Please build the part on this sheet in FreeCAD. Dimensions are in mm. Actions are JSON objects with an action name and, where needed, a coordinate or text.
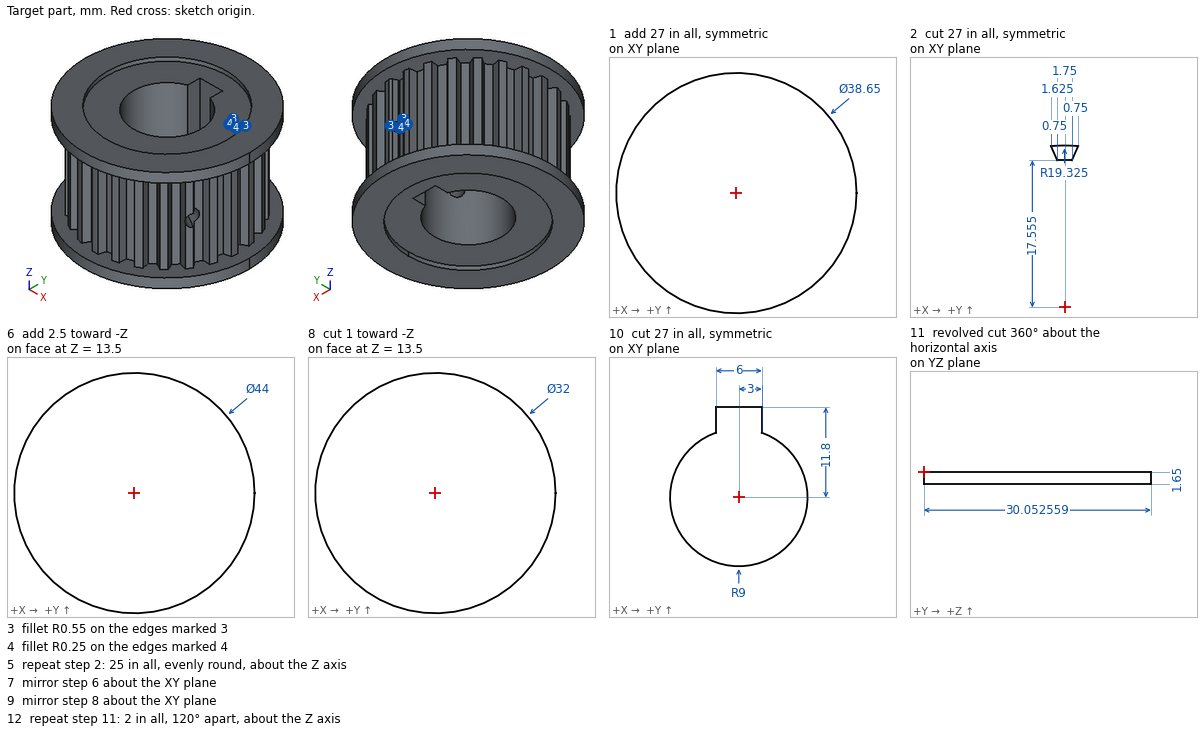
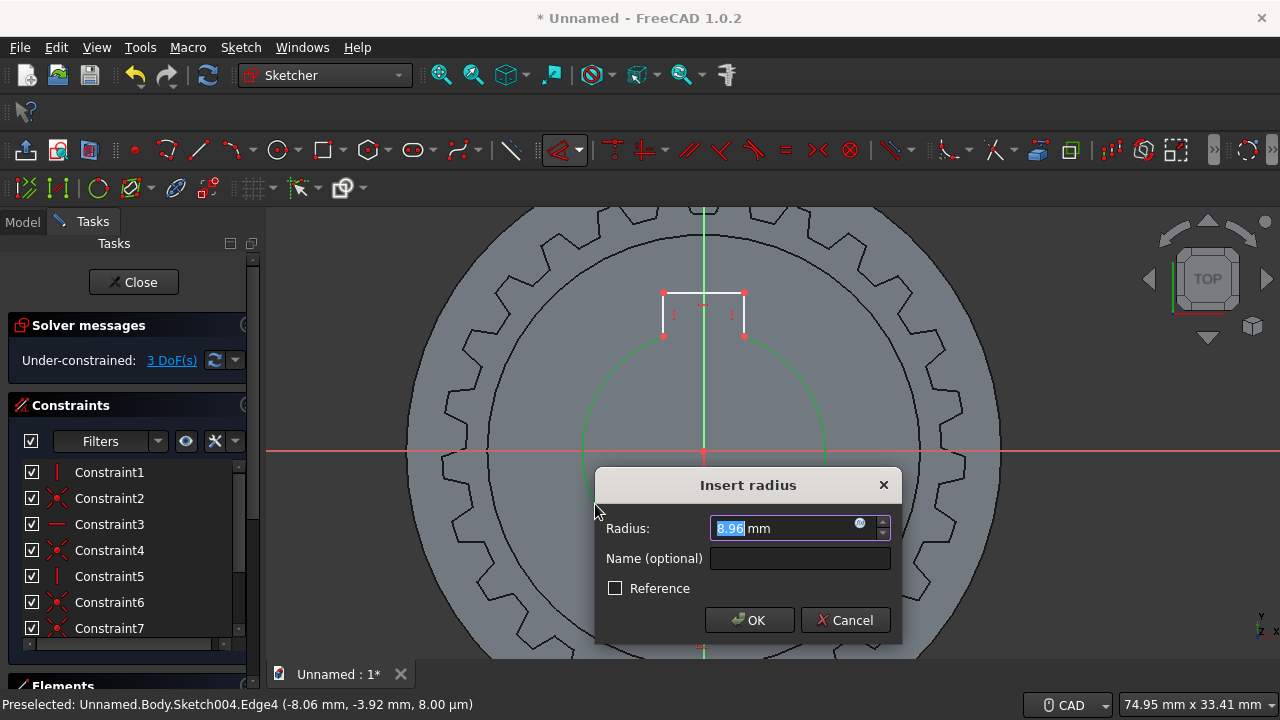
{"action": "type", "text": "9"}
{"action": "key", "text": "Return"}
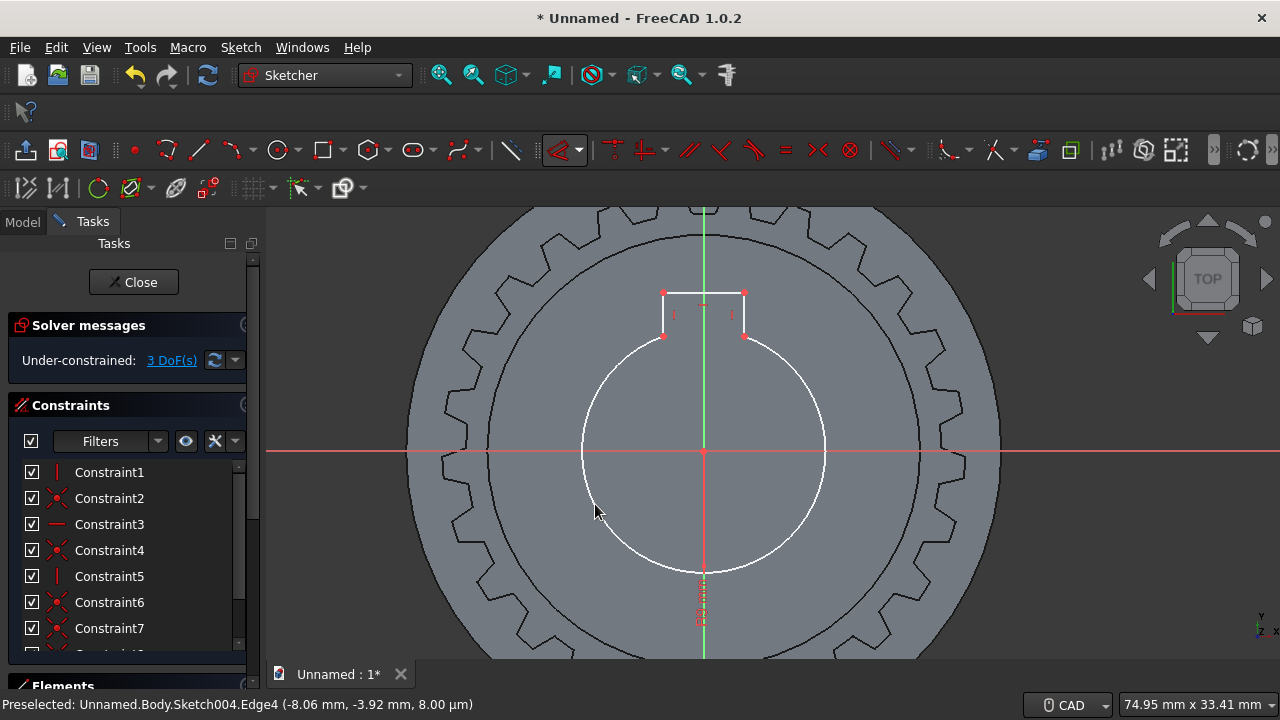
{"action": "left_click", "coordinate": [720, 293]}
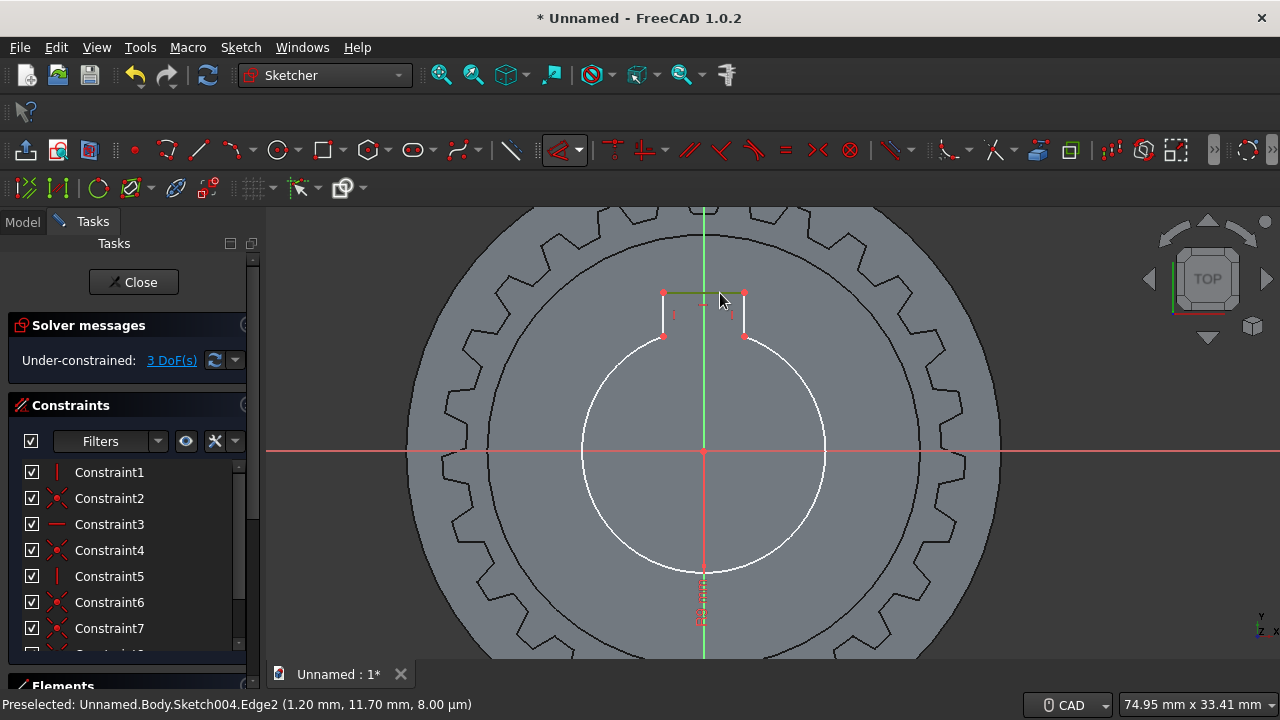
{"action": "left_click", "coordinate": [582, 150]}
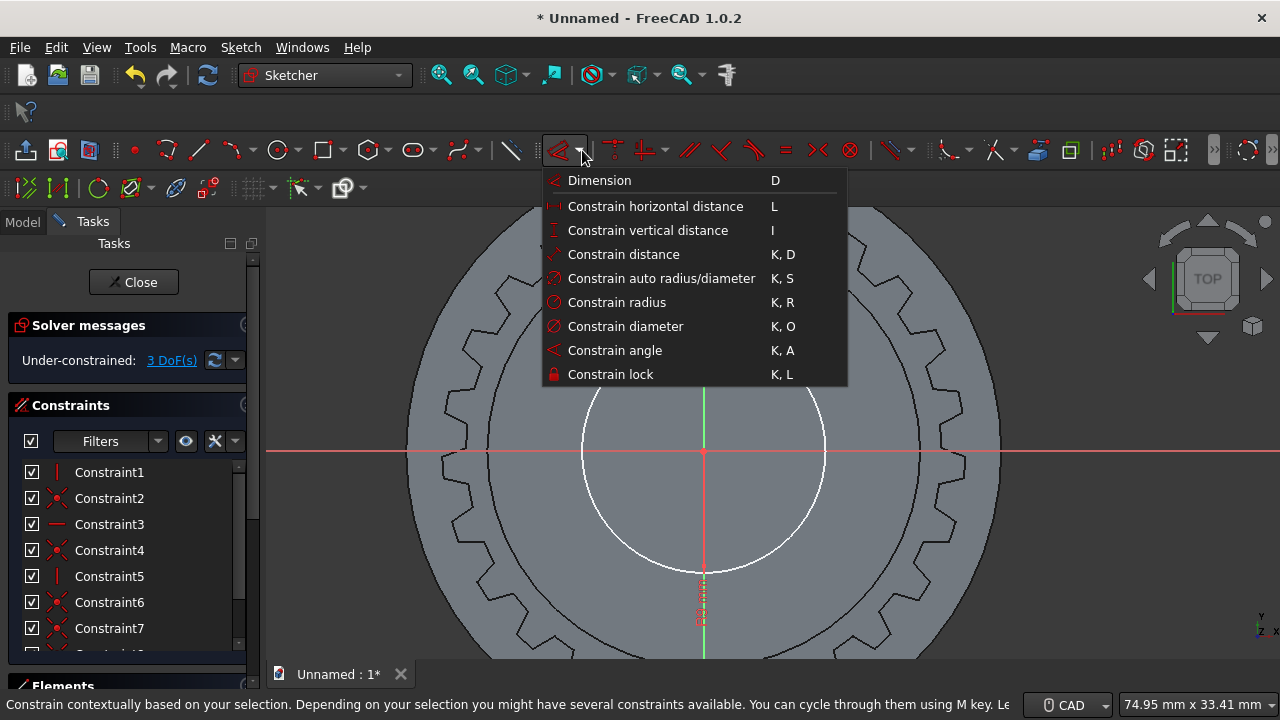
{"action": "left_click", "coordinate": [695, 206]}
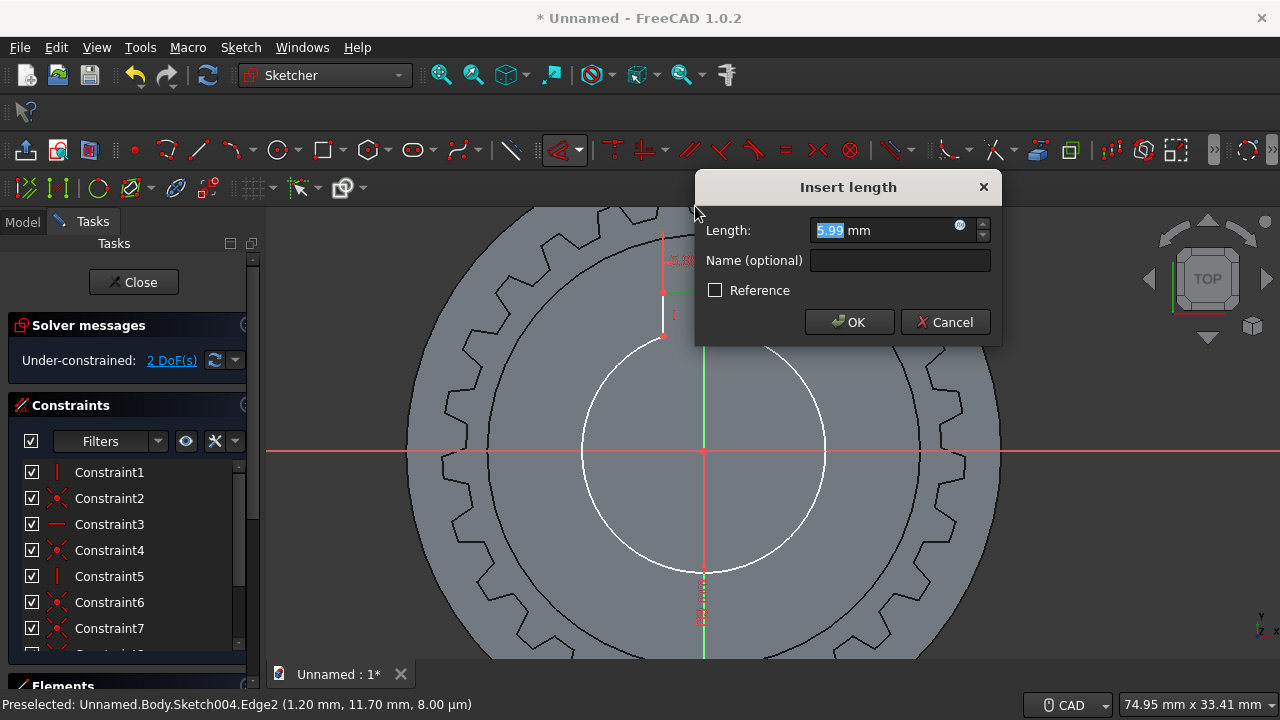
{"action": "type", "text": "6"}
{"action": "key", "text": "Return"}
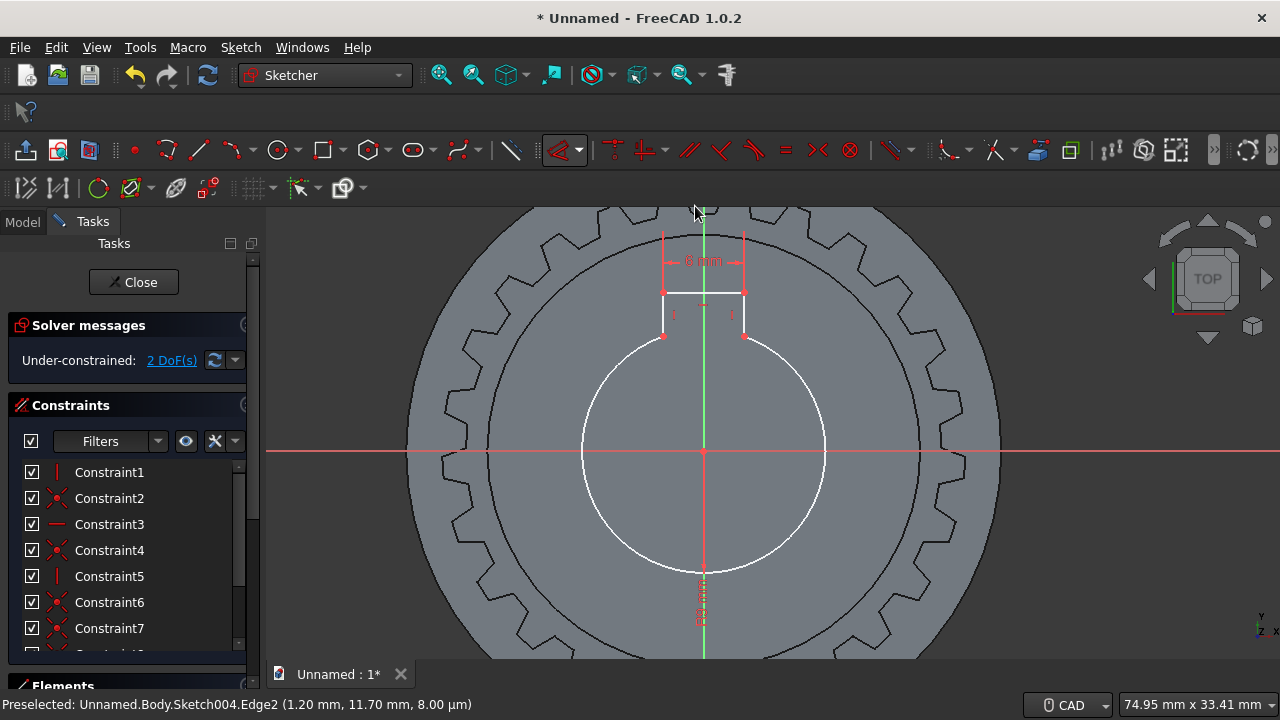
{"action": "left_click", "coordinate": [744, 336]}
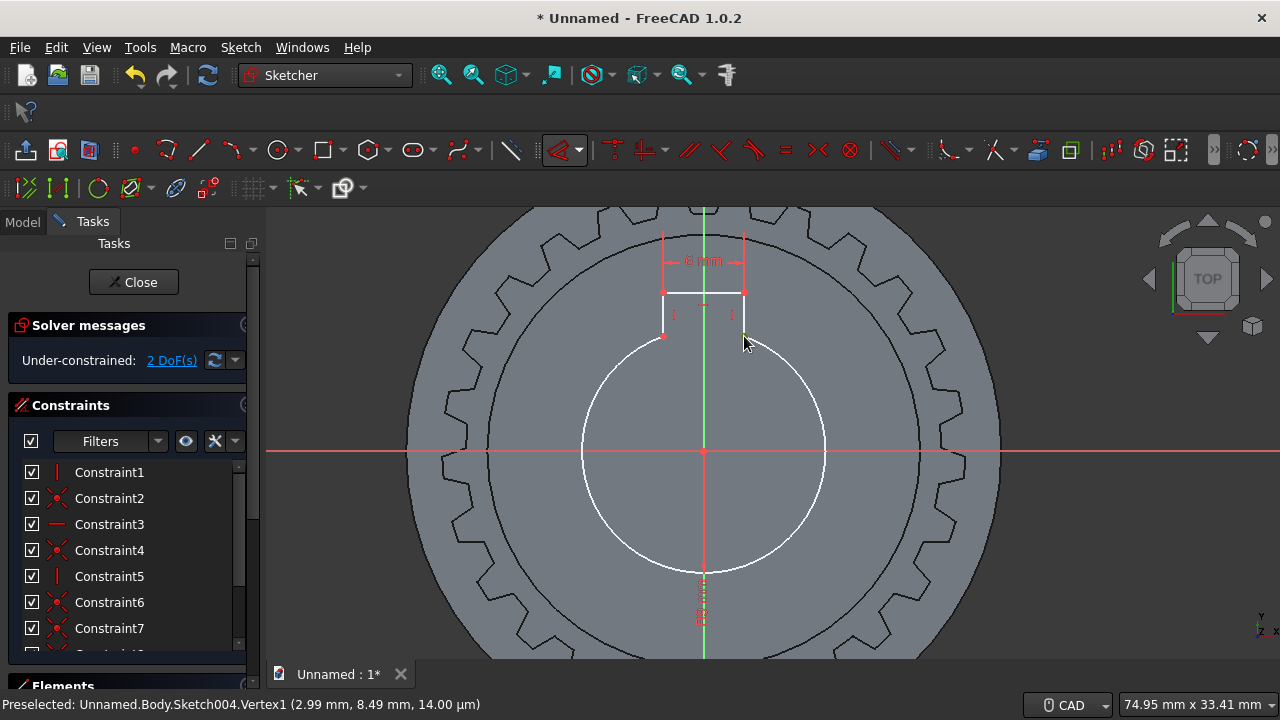
{"action": "left_click", "coordinate": [582, 150]}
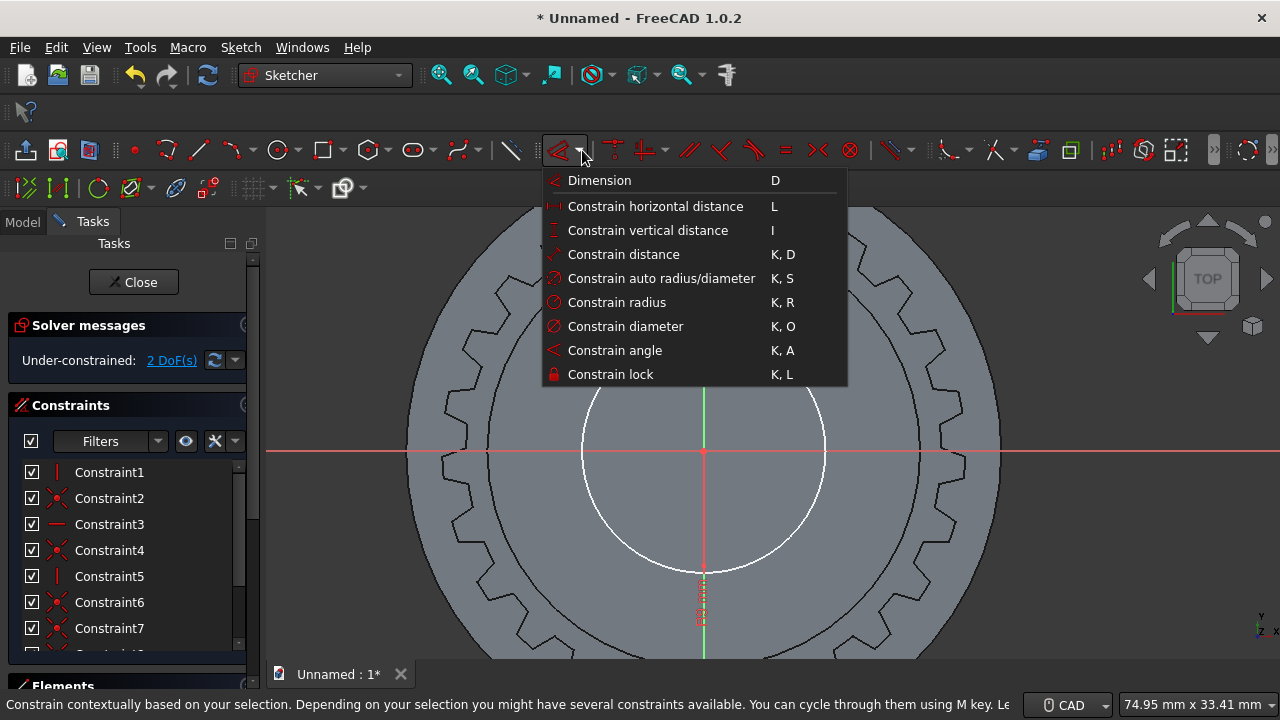
{"action": "left_click", "coordinate": [695, 206]}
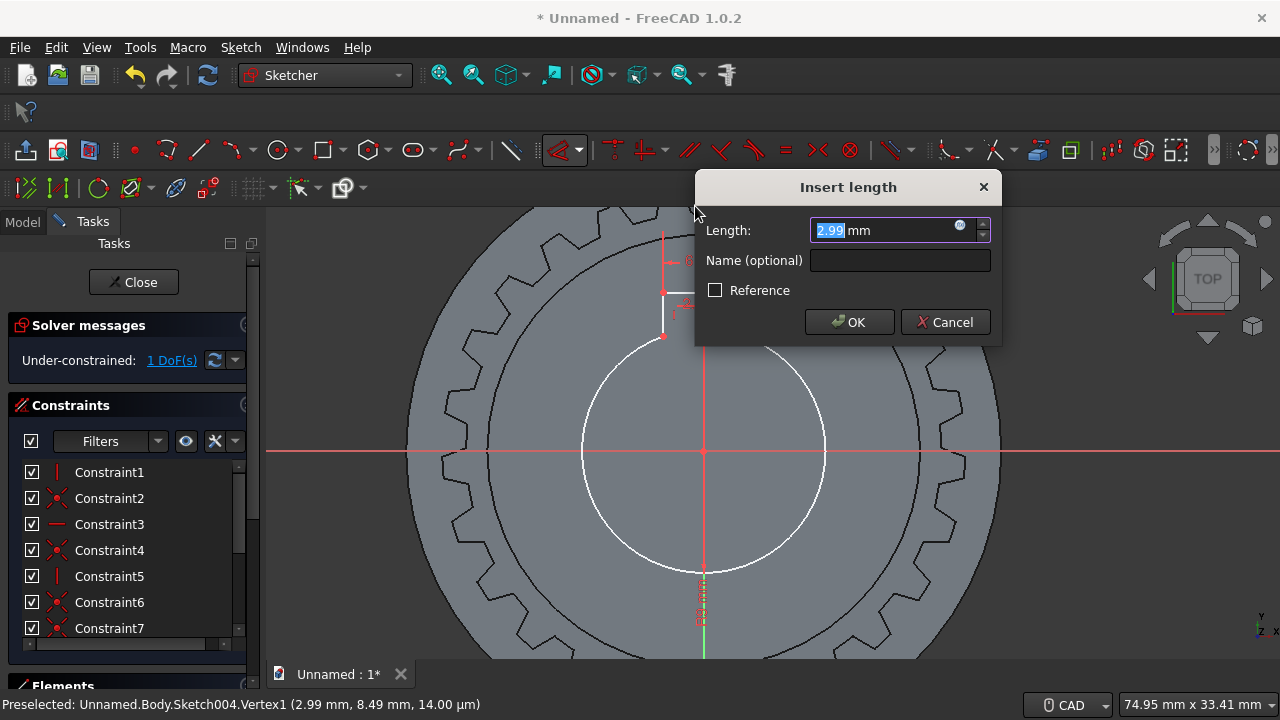
{"action": "type", "text": "3"}
{"action": "key", "text": "Return"}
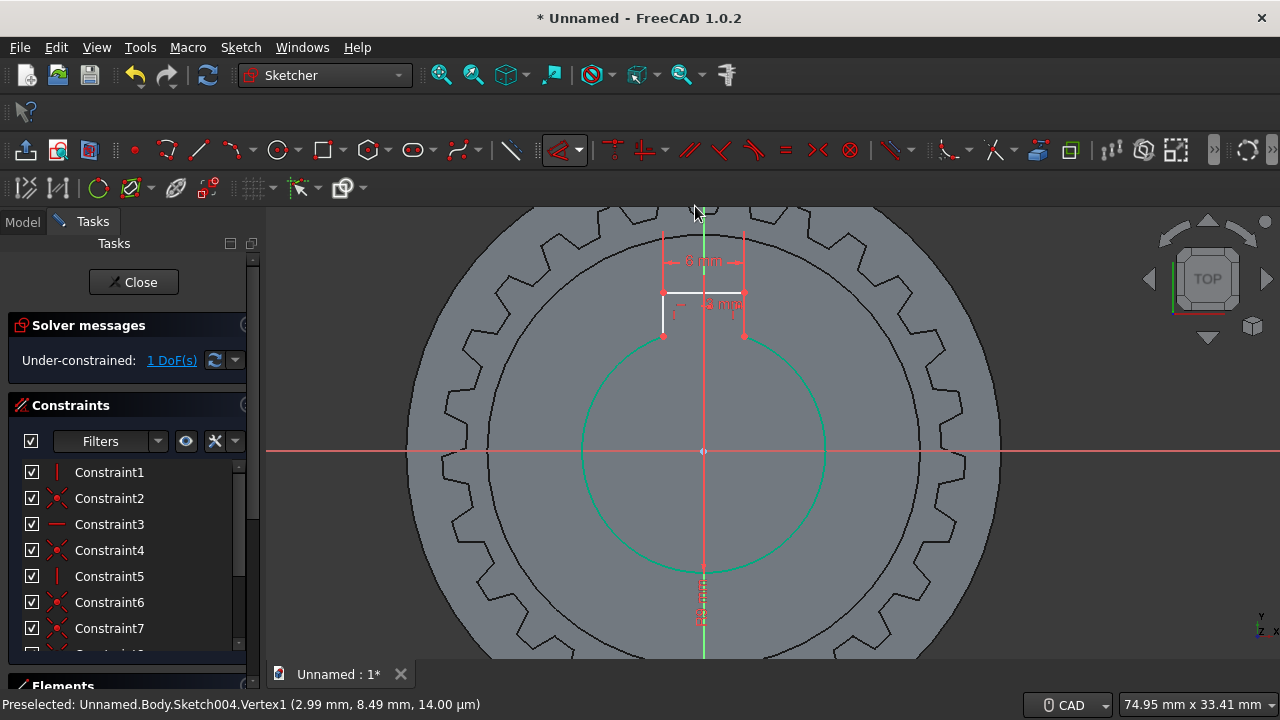
{"action": "left_click", "coordinate": [744, 293]}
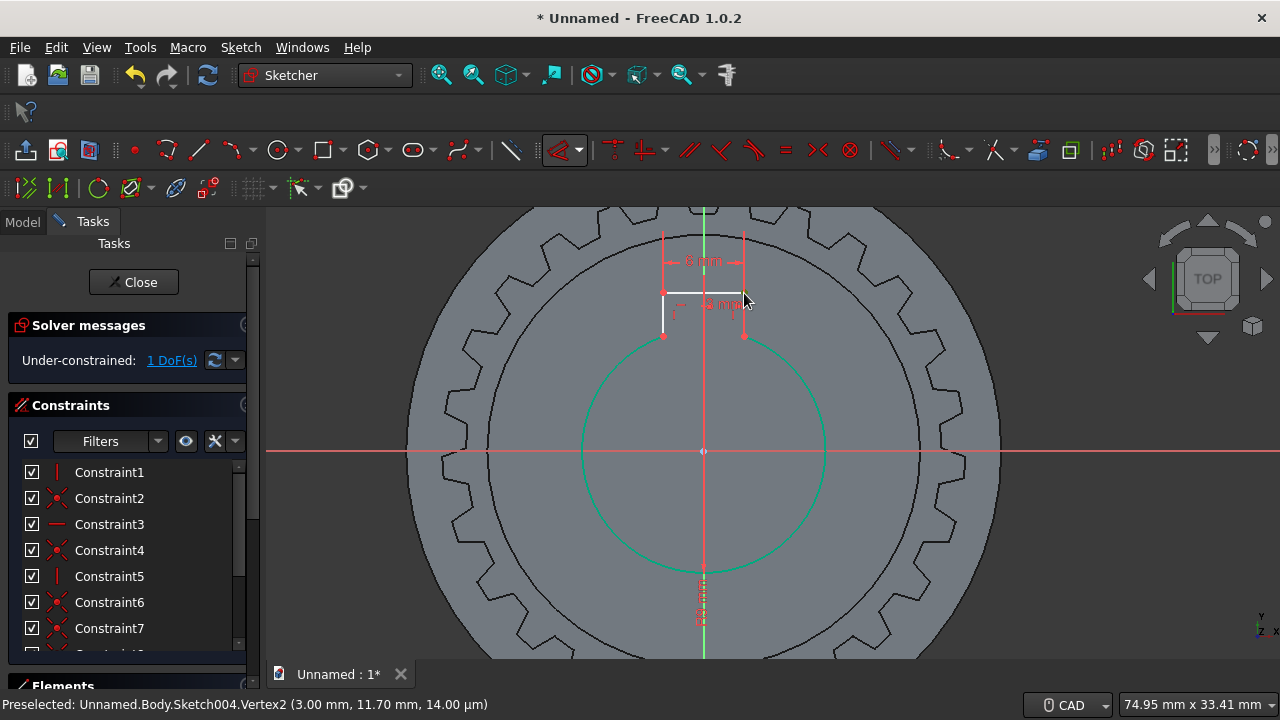
{"action": "key", "text": "i"}